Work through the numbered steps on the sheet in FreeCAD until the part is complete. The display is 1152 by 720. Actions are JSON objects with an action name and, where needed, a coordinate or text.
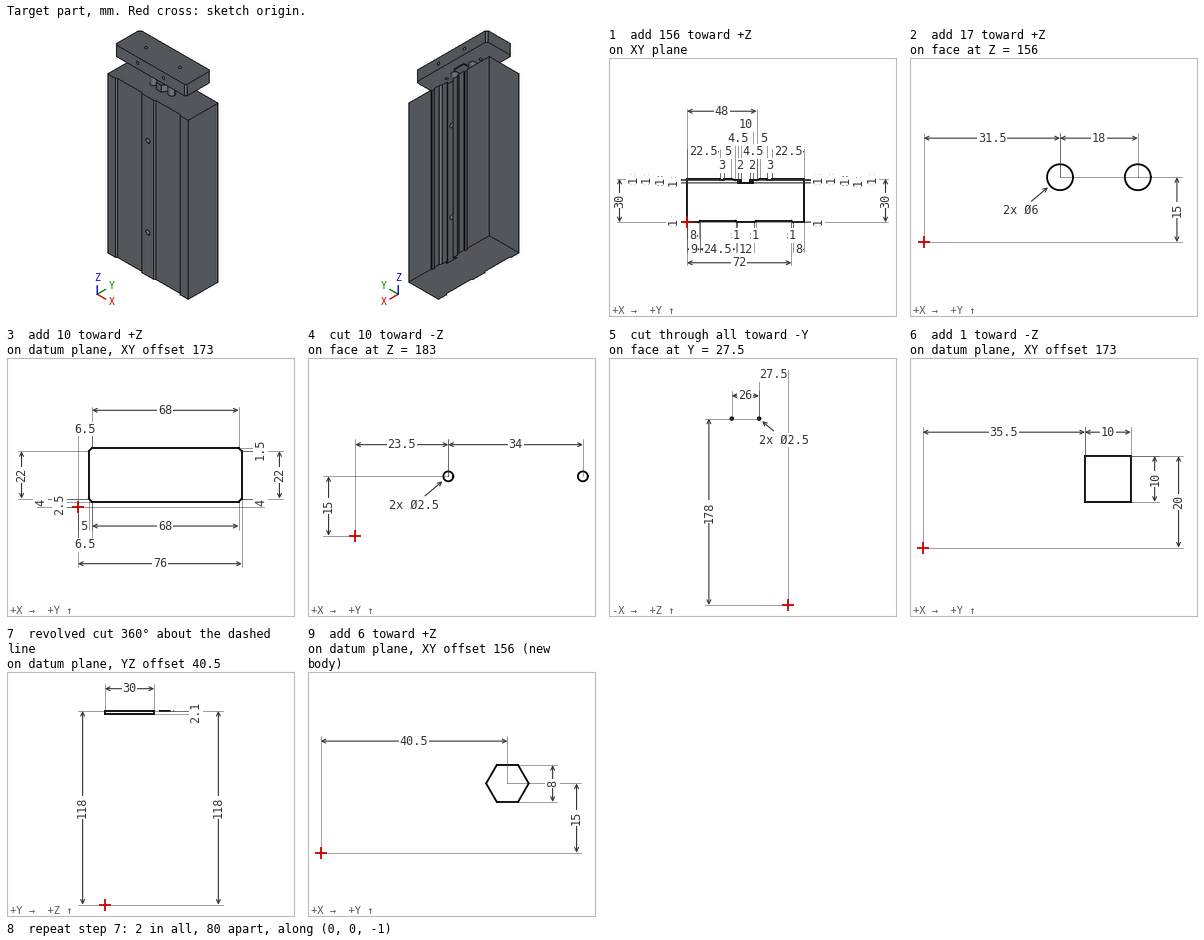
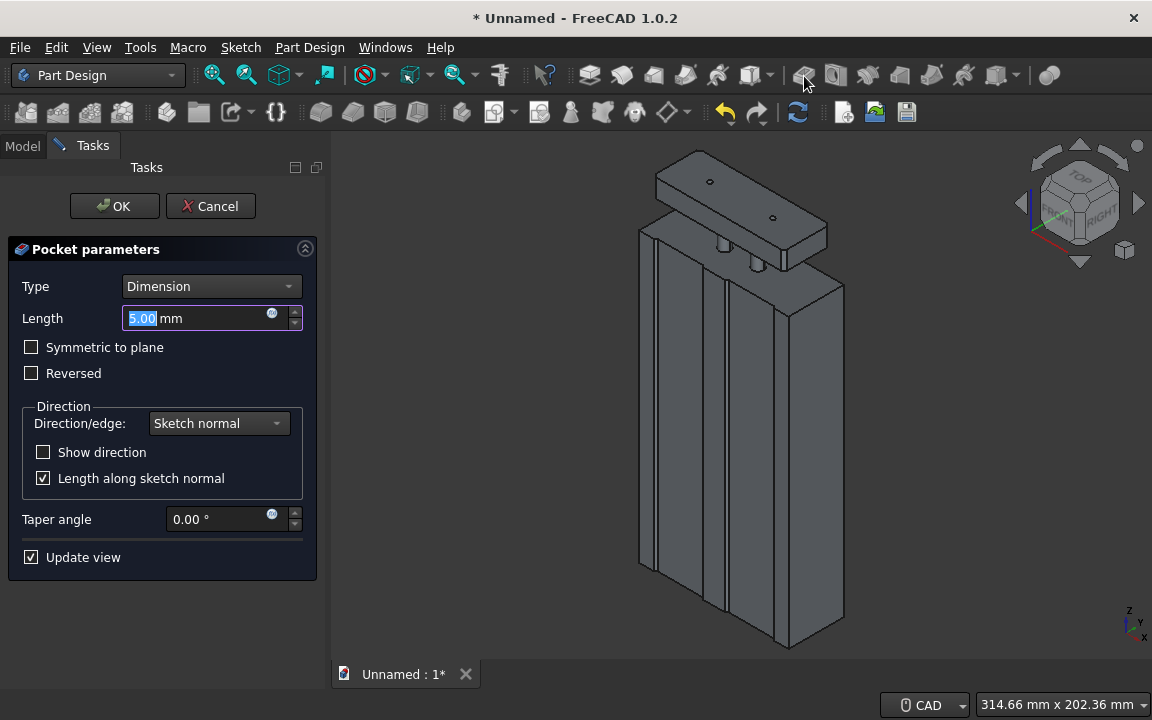
{"action": "type", "text": "10"}
{"action": "key", "text": "Tab"}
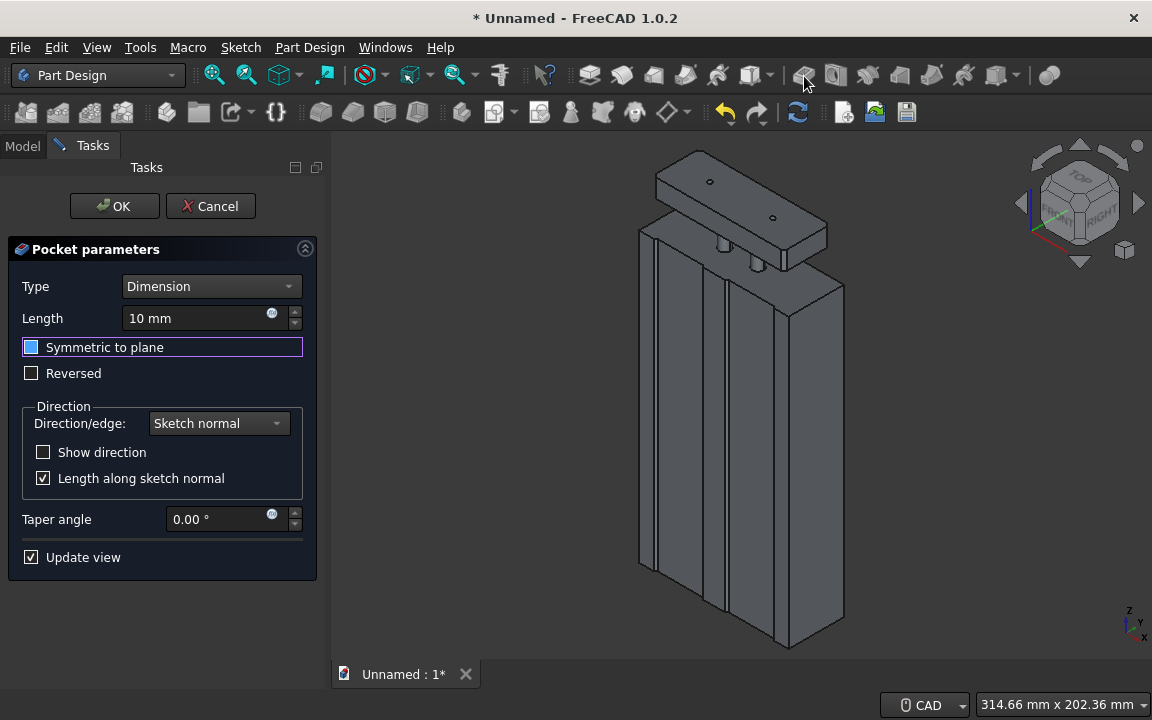
{"action": "left_click", "coordinate": [115, 206]}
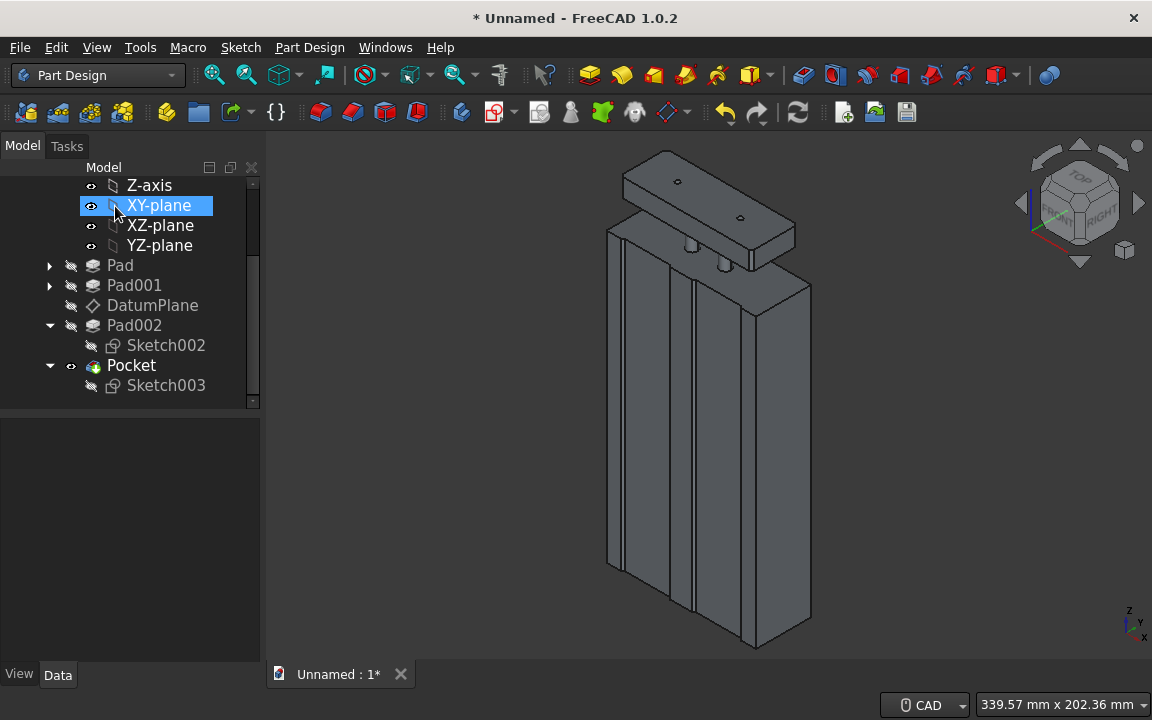
{"action": "key", "text": "4"}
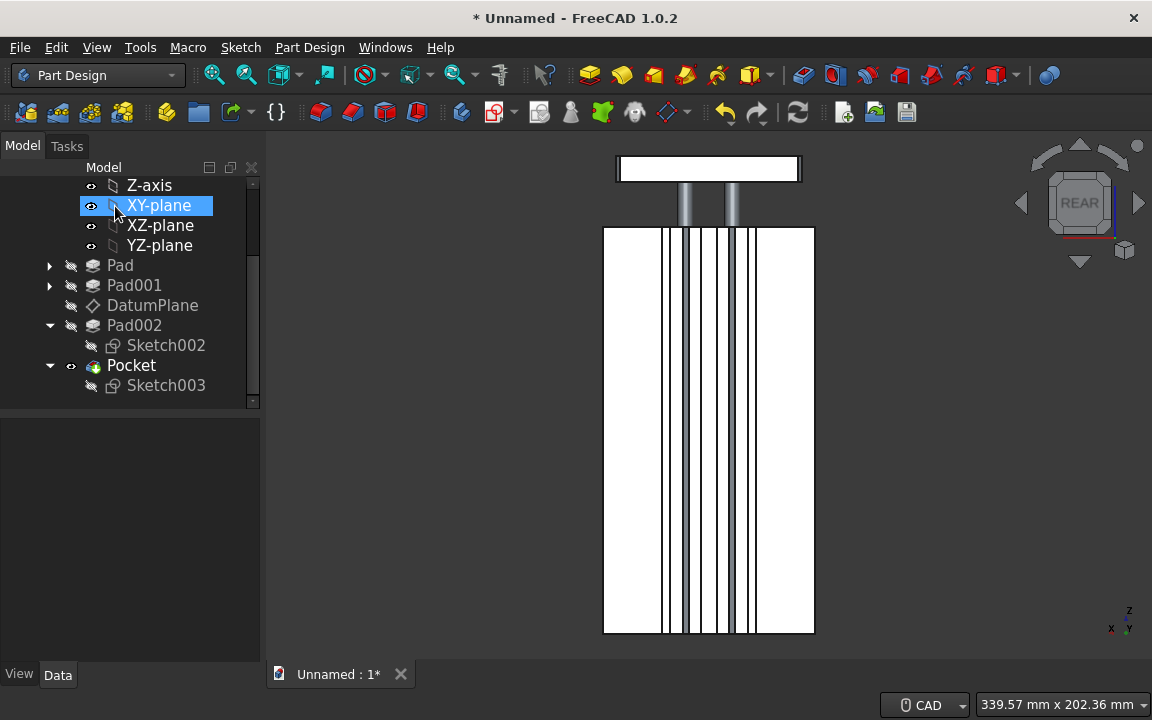
{"action": "left_click", "coordinate": [658, 168]}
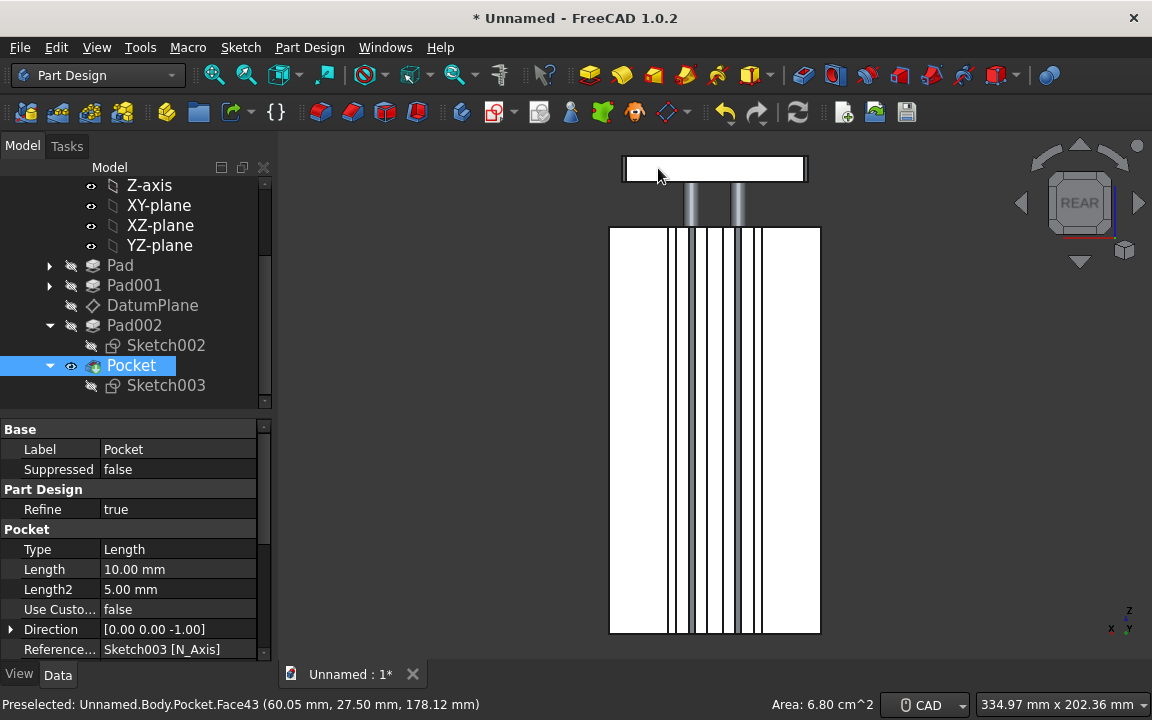
{"action": "left_click", "coordinate": [494, 112]}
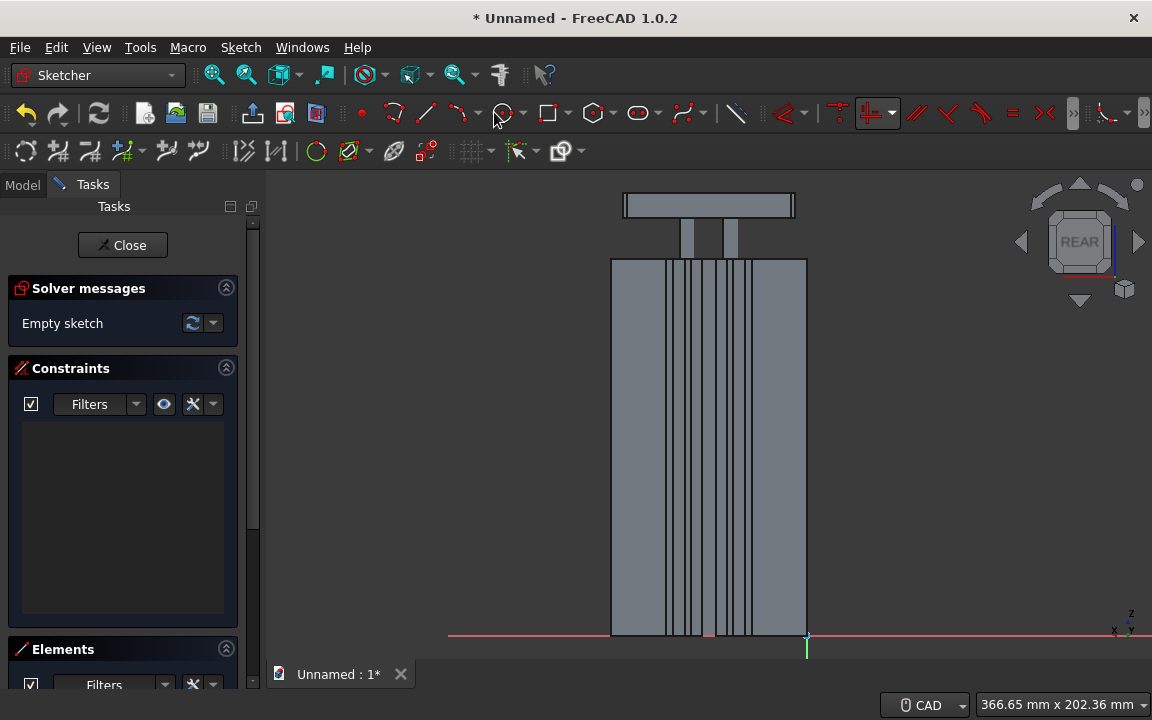
{"action": "left_click", "coordinate": [318, 114]}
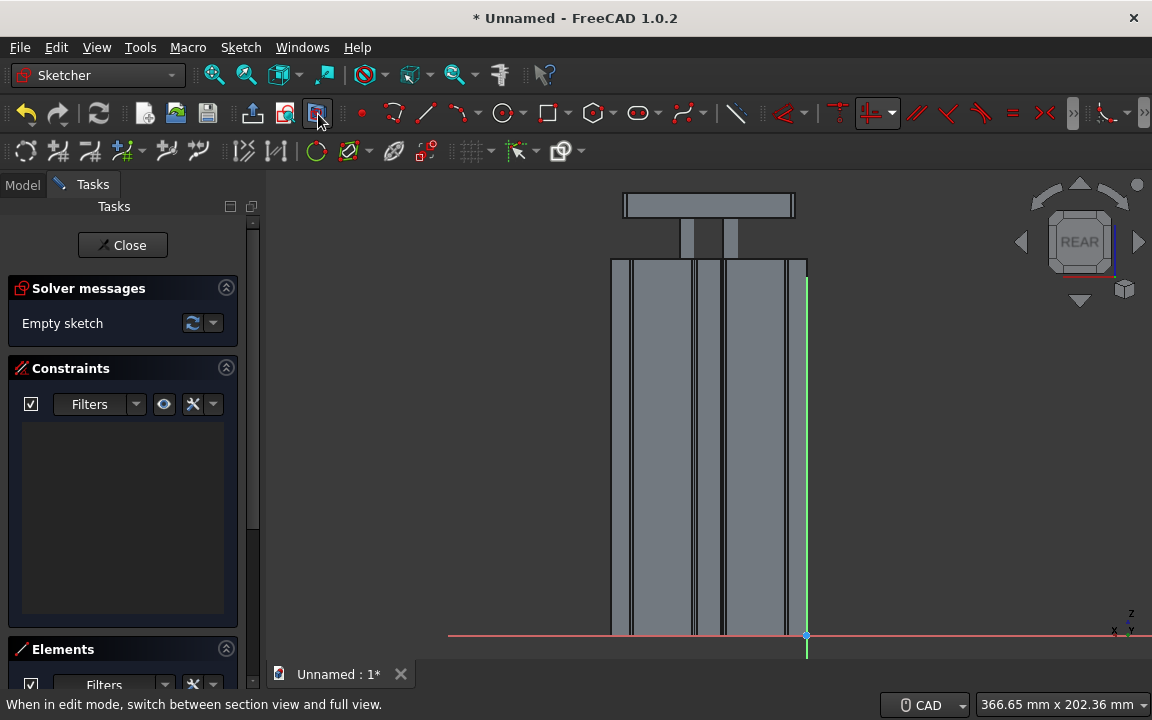
{"action": "scroll", "coordinate": [720, 198], "scroll_direction": "up", "scroll_amount": 10}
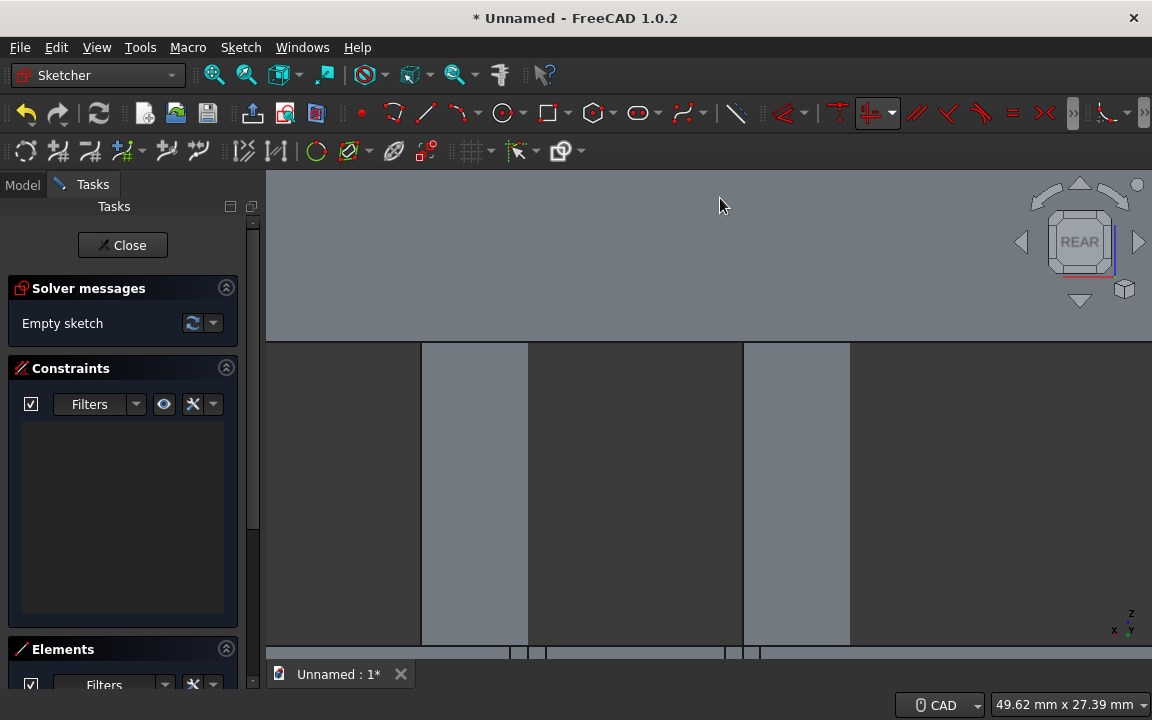
{"action": "key", "text": "g c"}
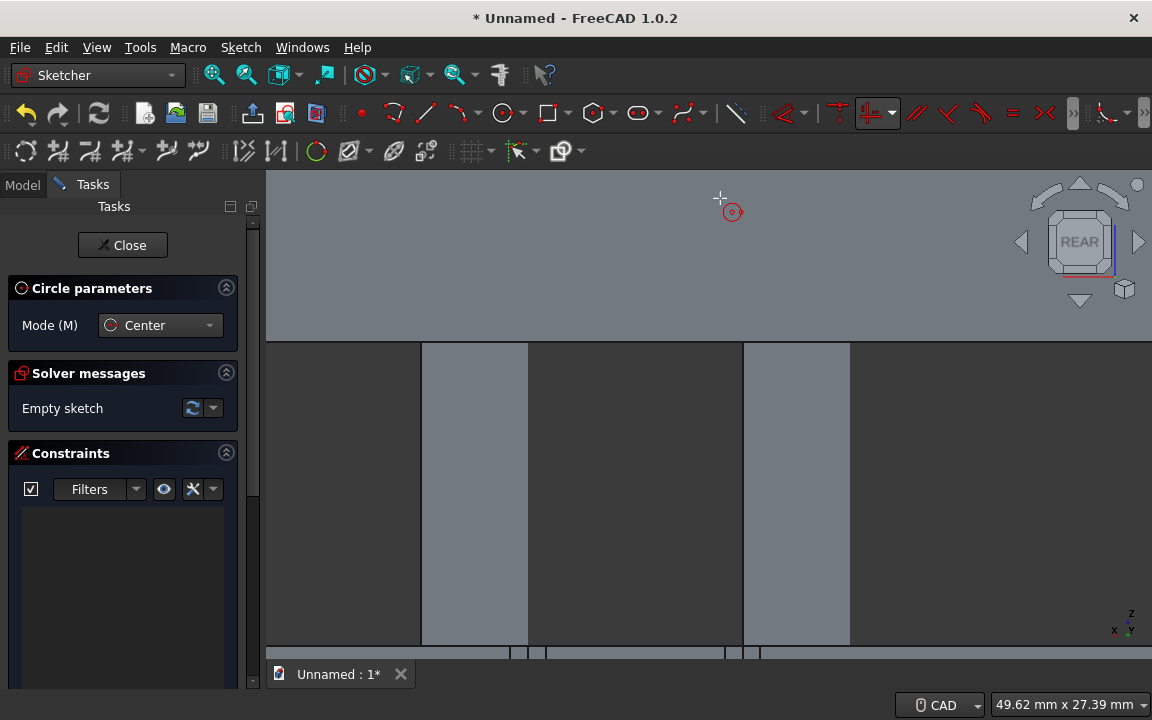
{"action": "left_click", "coordinate": [868, 253]}
{"action": "mouse_move", "coordinate": [883, 237]}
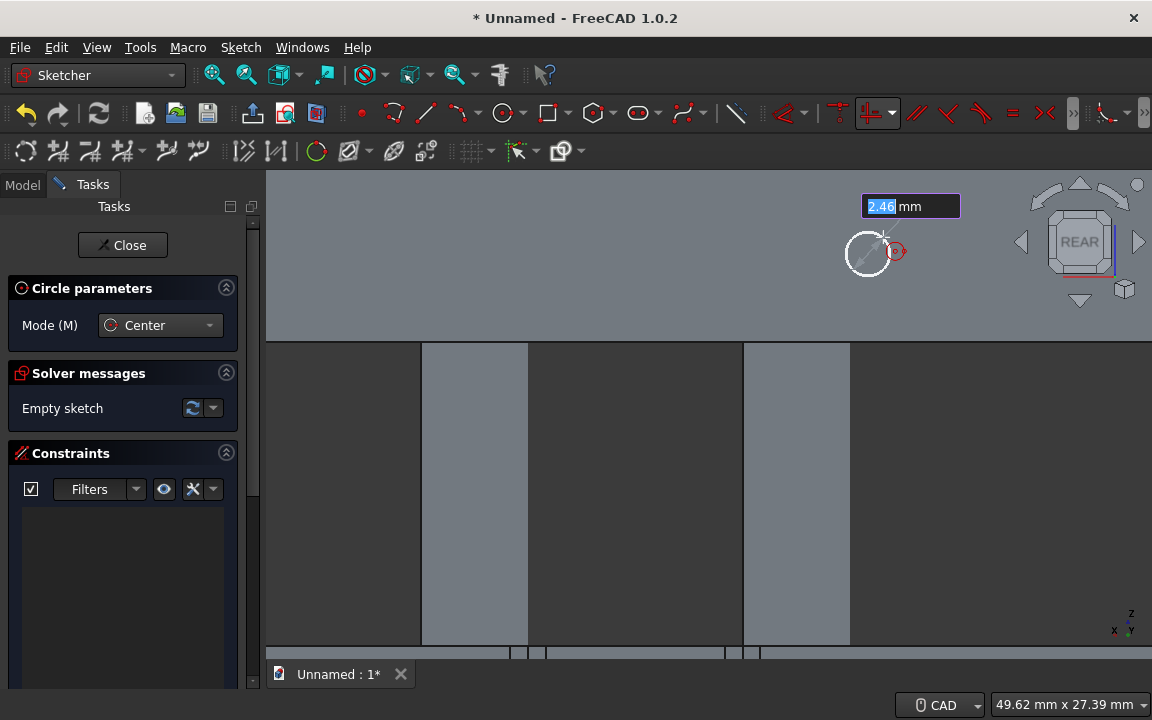
{"action": "type", "text": "2.5"}
{"action": "key", "text": "Return"}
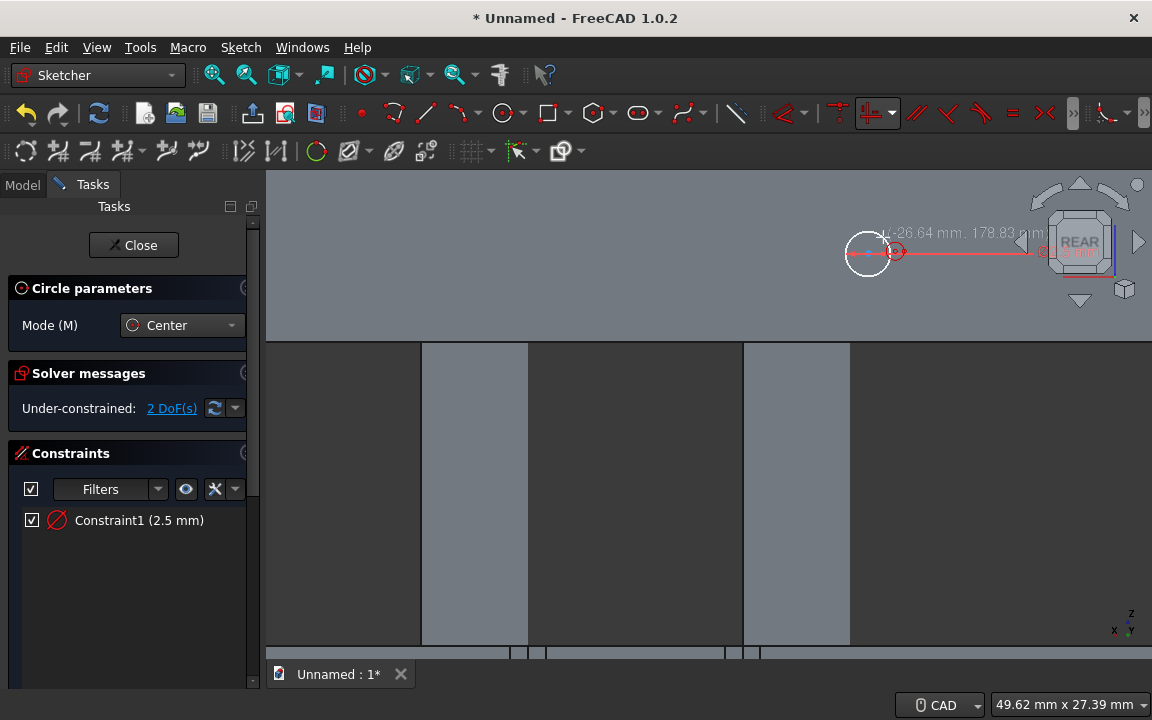
{"action": "left_click", "coordinate": [403, 253]}
{"action": "mouse_move", "coordinate": [419, 237]}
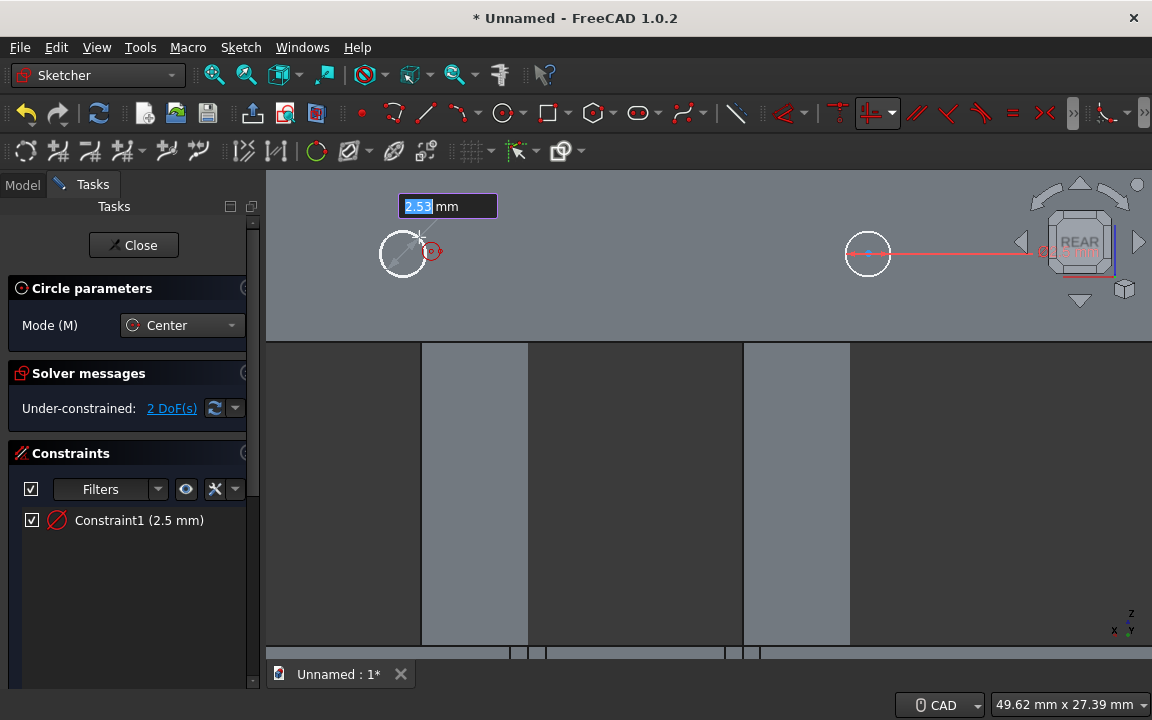
{"action": "type", "text": "2.5"}
{"action": "key", "text": "Return"}
{"action": "key", "text": "Escape"}